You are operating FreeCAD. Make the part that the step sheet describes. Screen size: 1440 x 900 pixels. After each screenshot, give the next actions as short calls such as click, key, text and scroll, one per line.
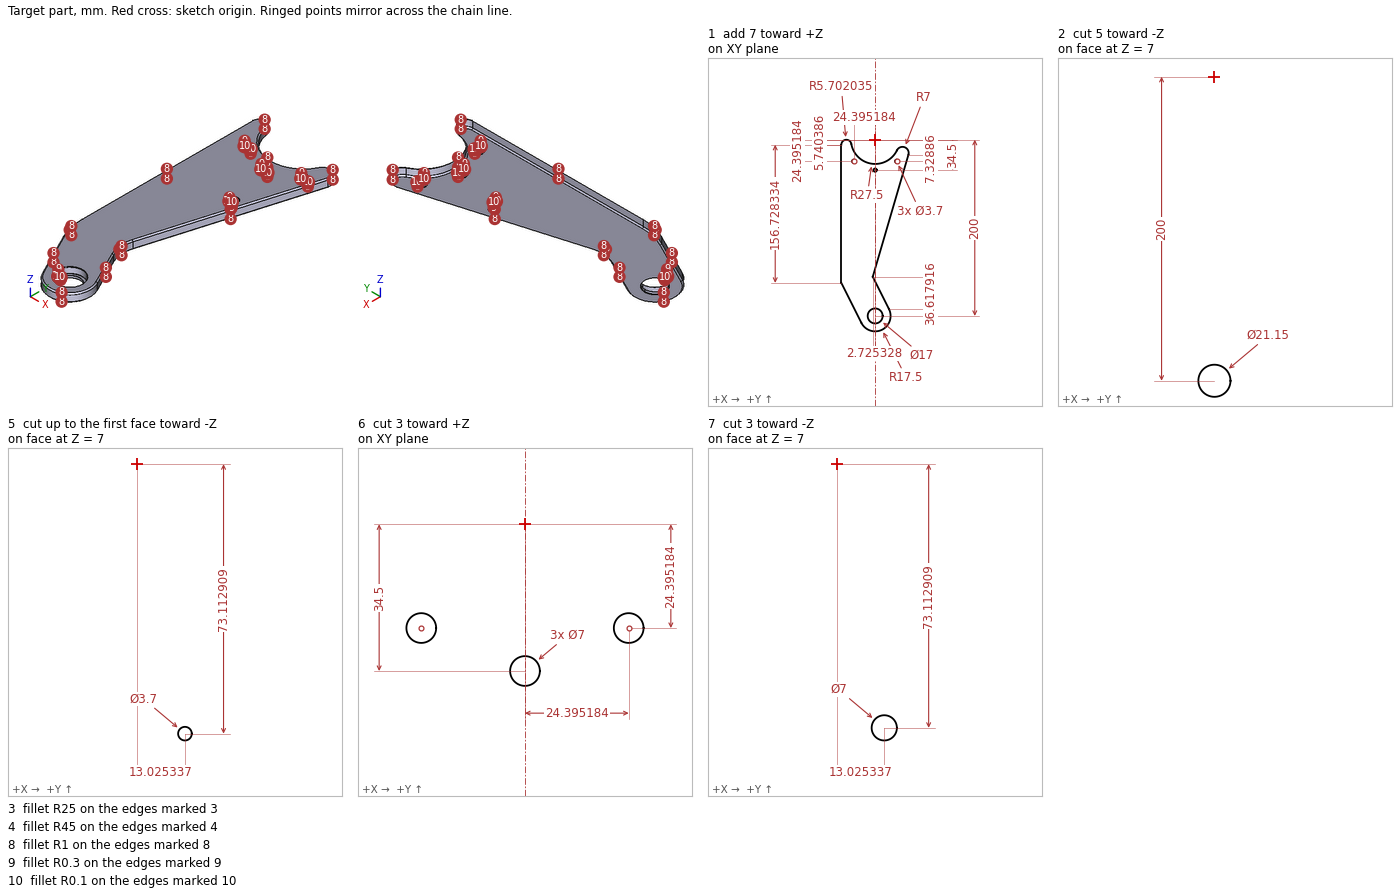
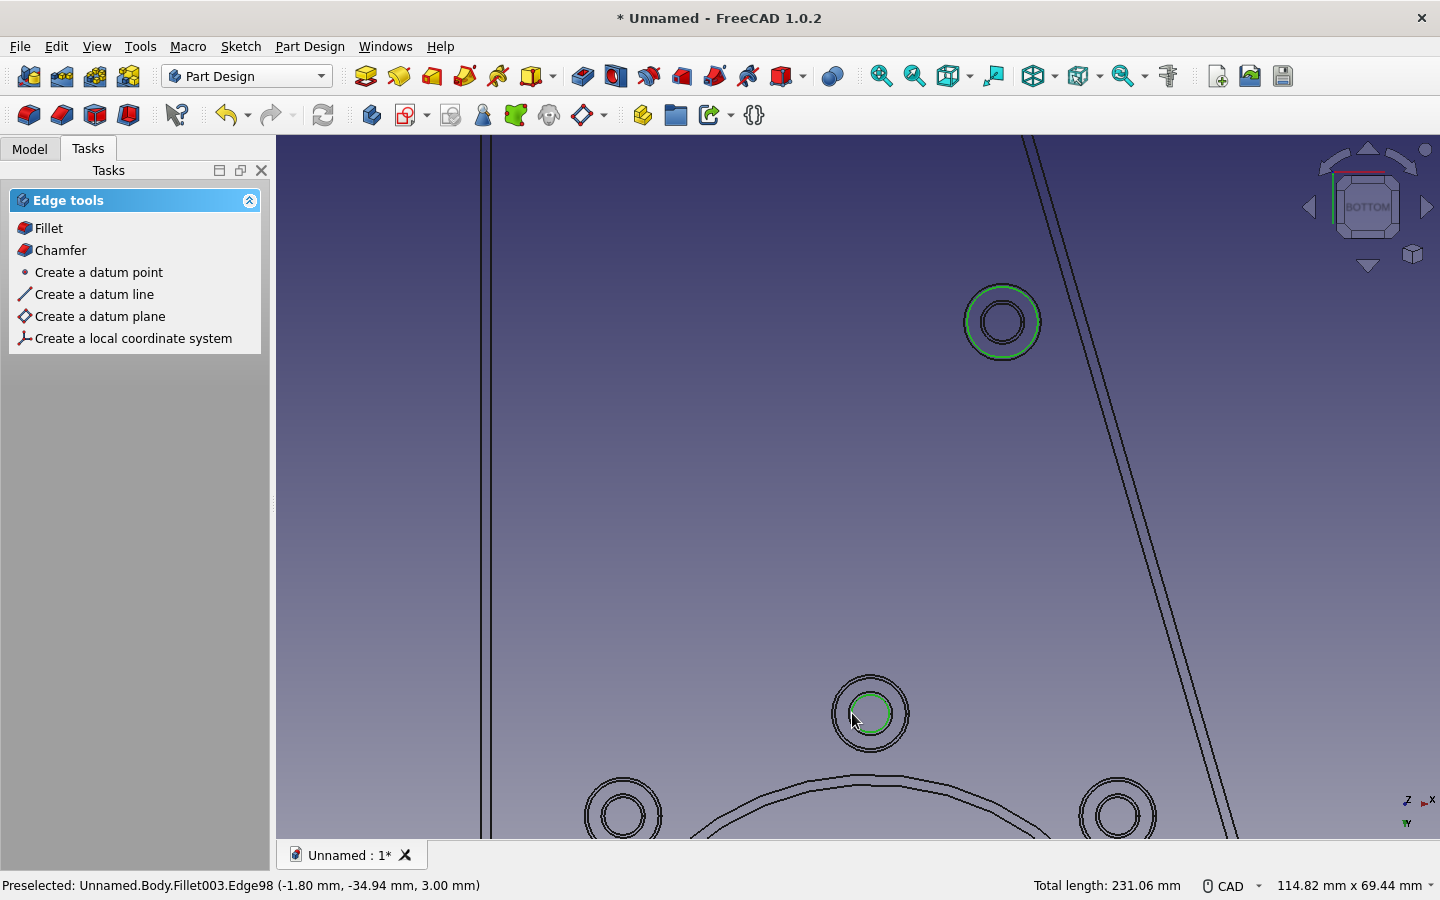
click(1103, 804, ctrl)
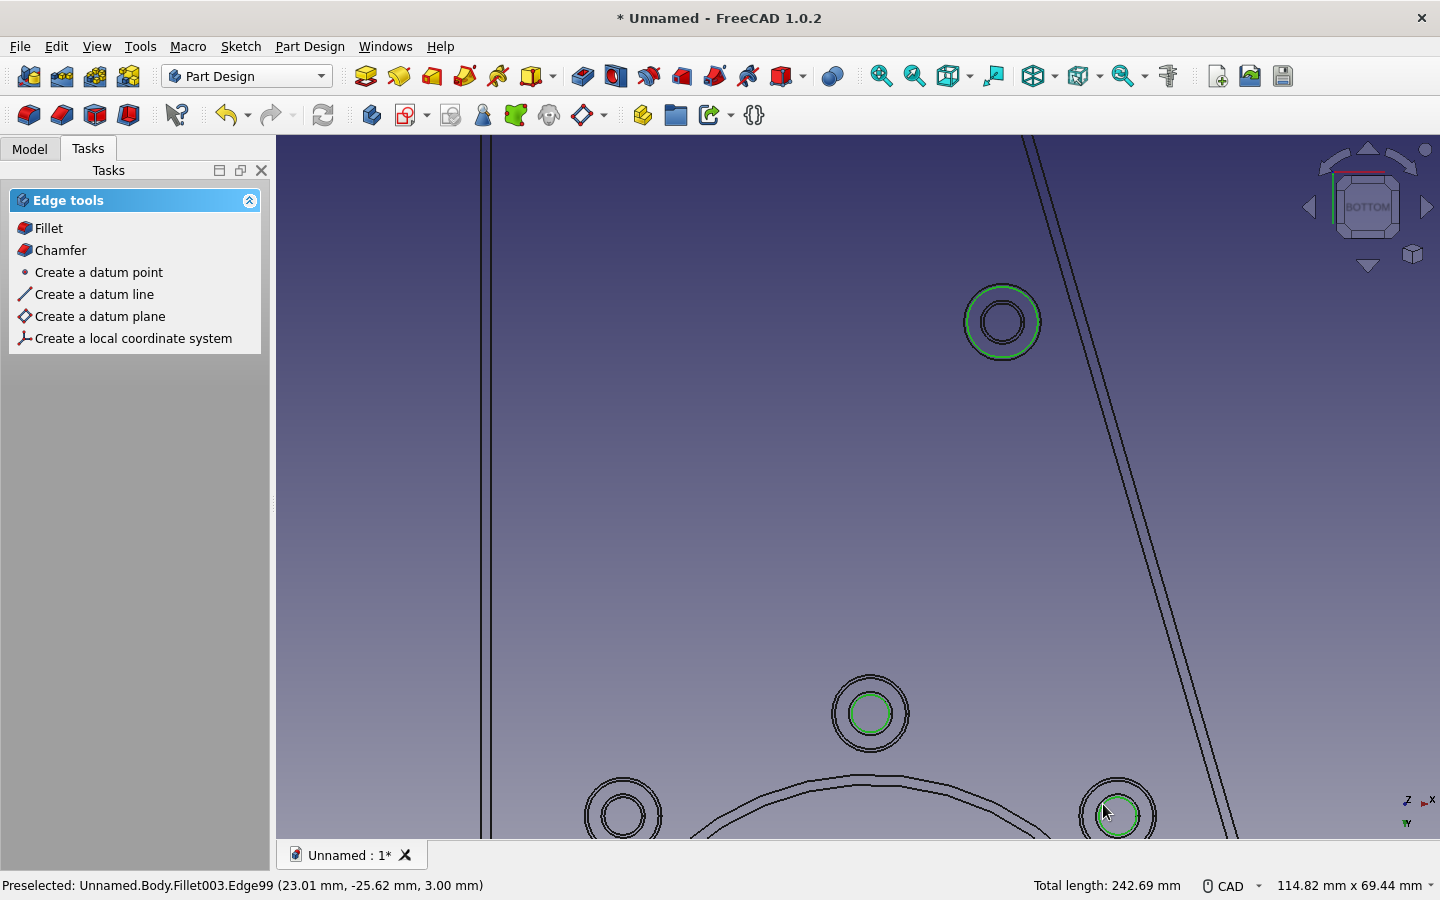
click(608, 804, ctrl)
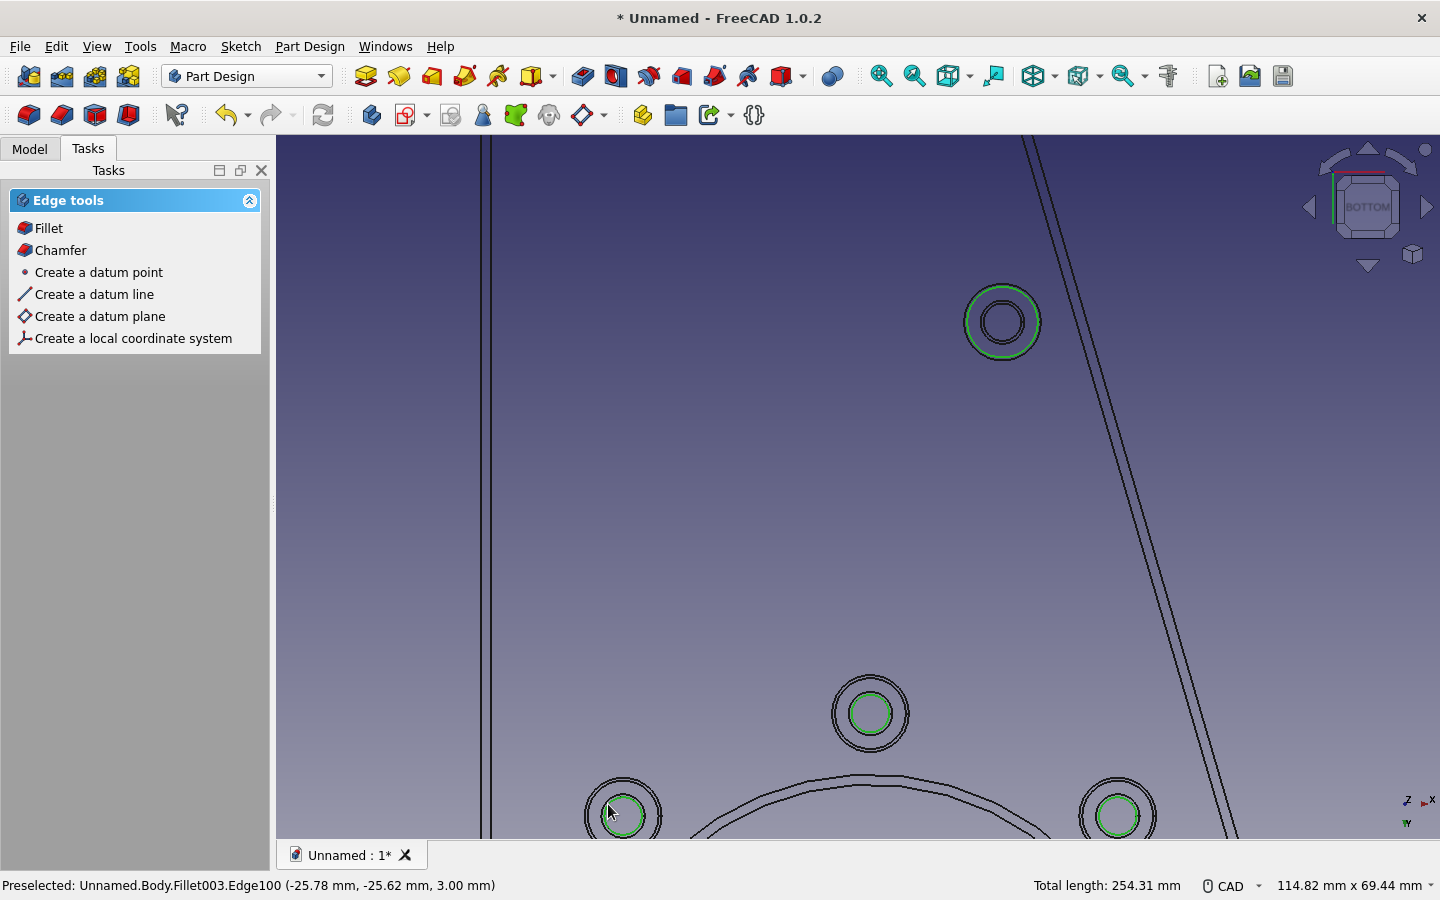
key(v)
key(1)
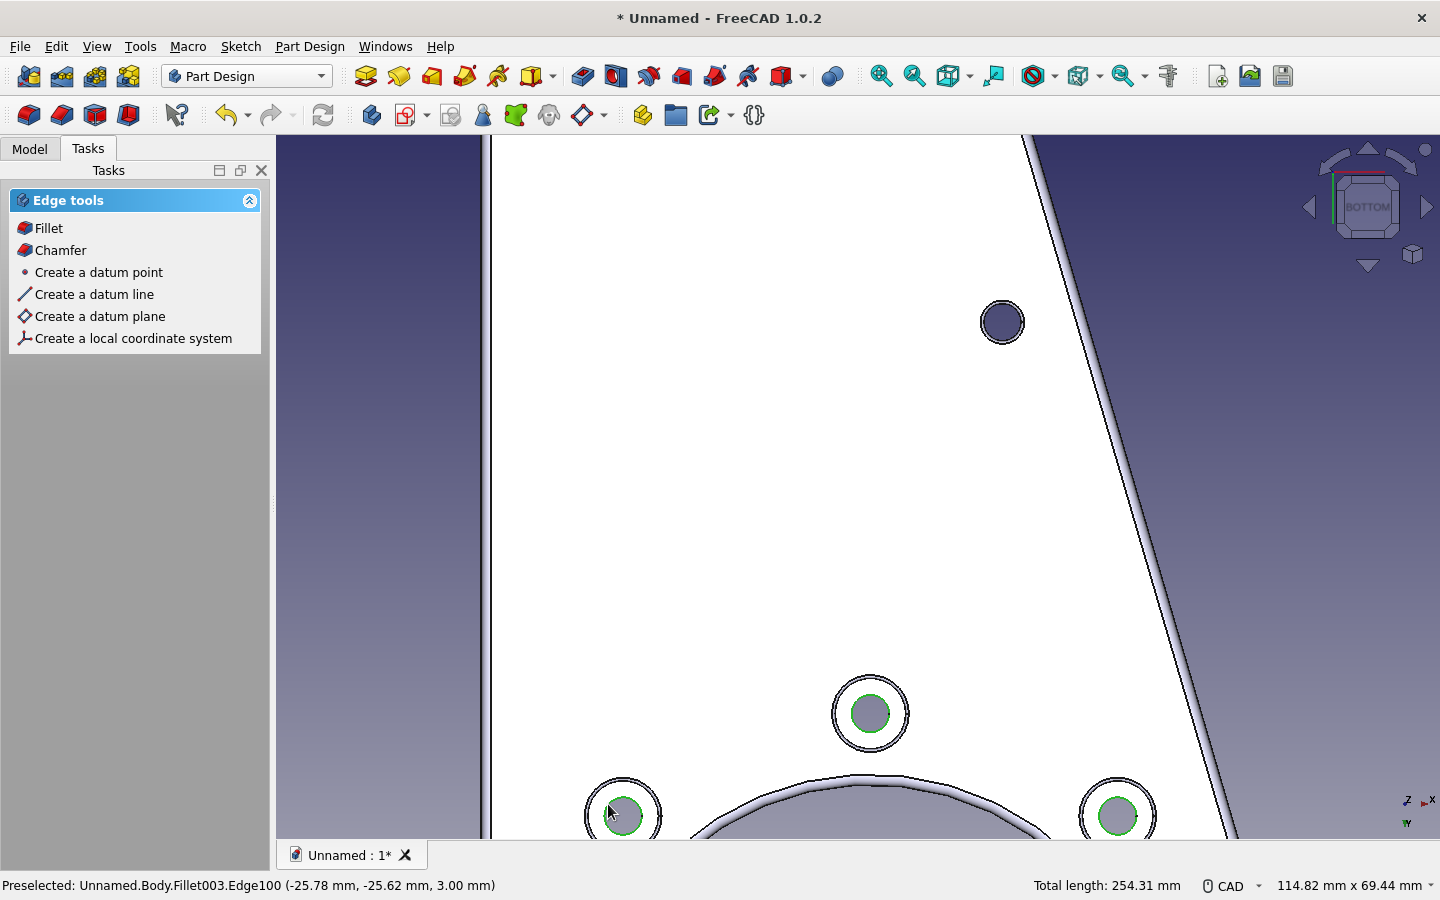
click(29, 116)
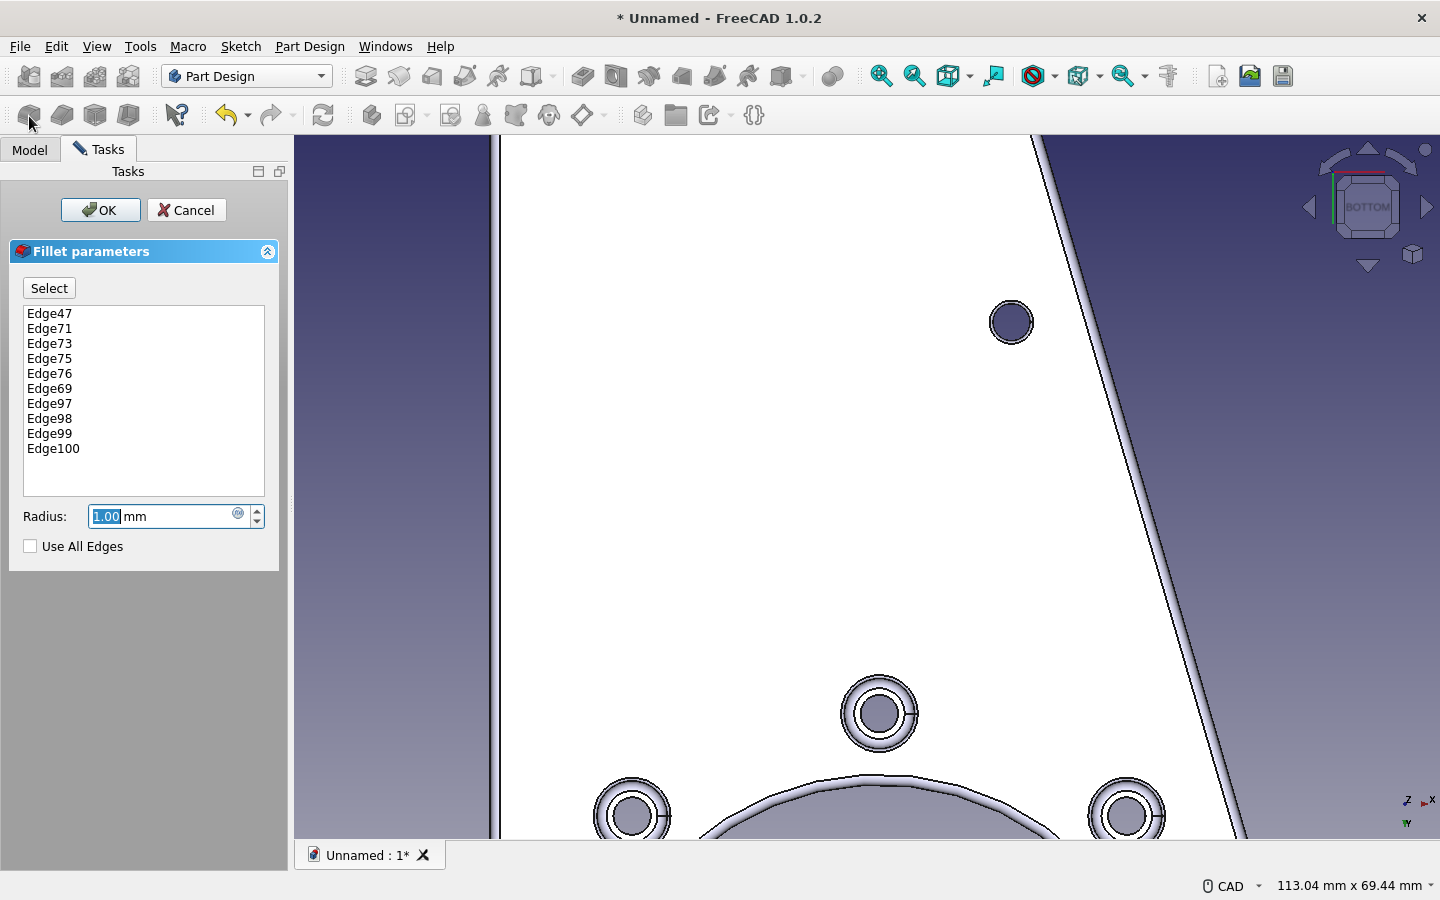
text(0.1)
key(Tab)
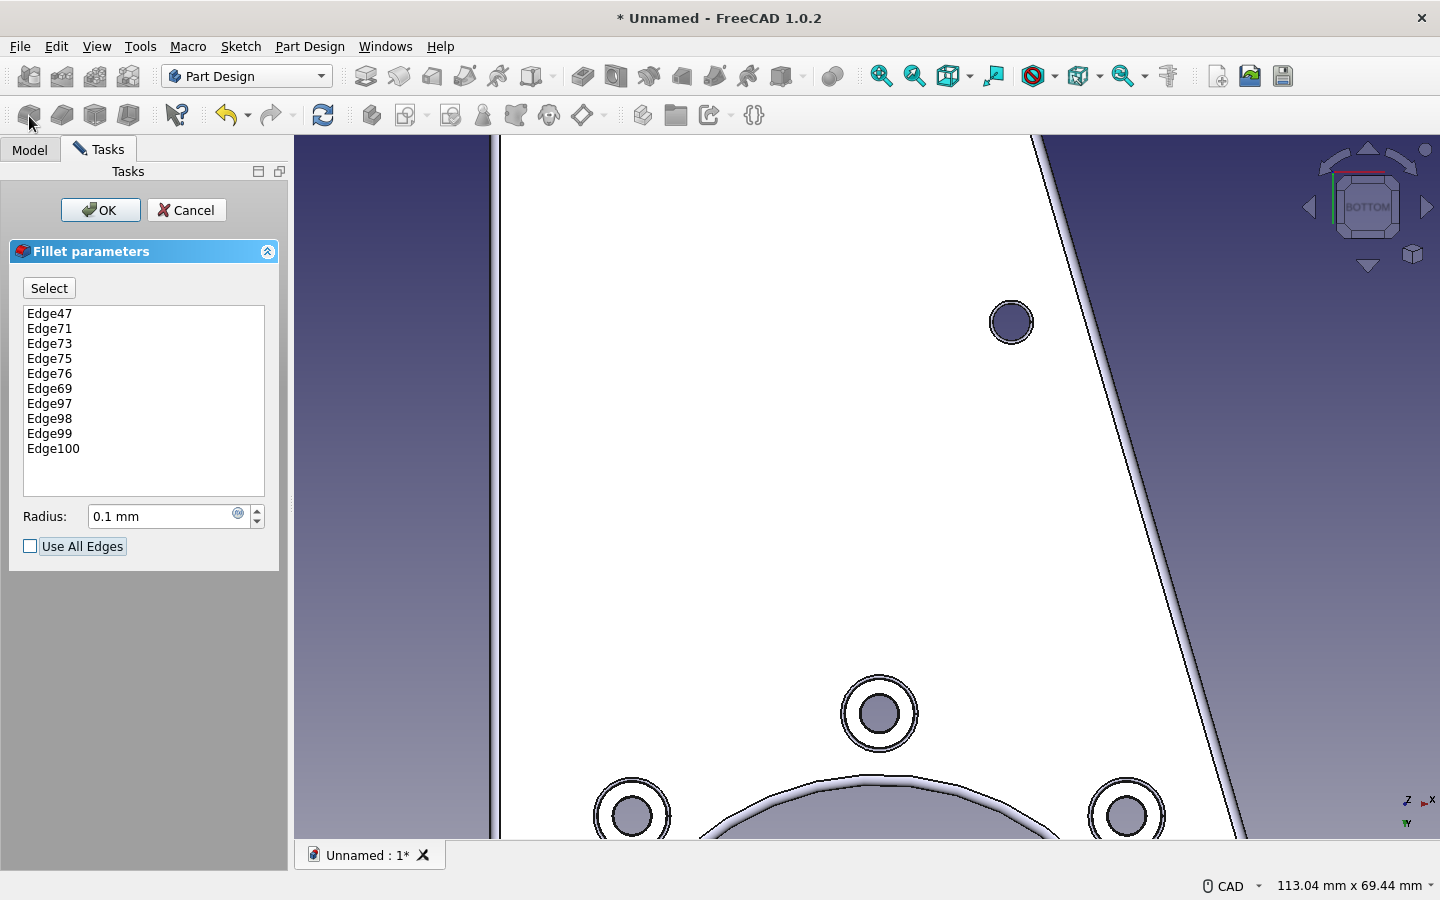
click(101, 210)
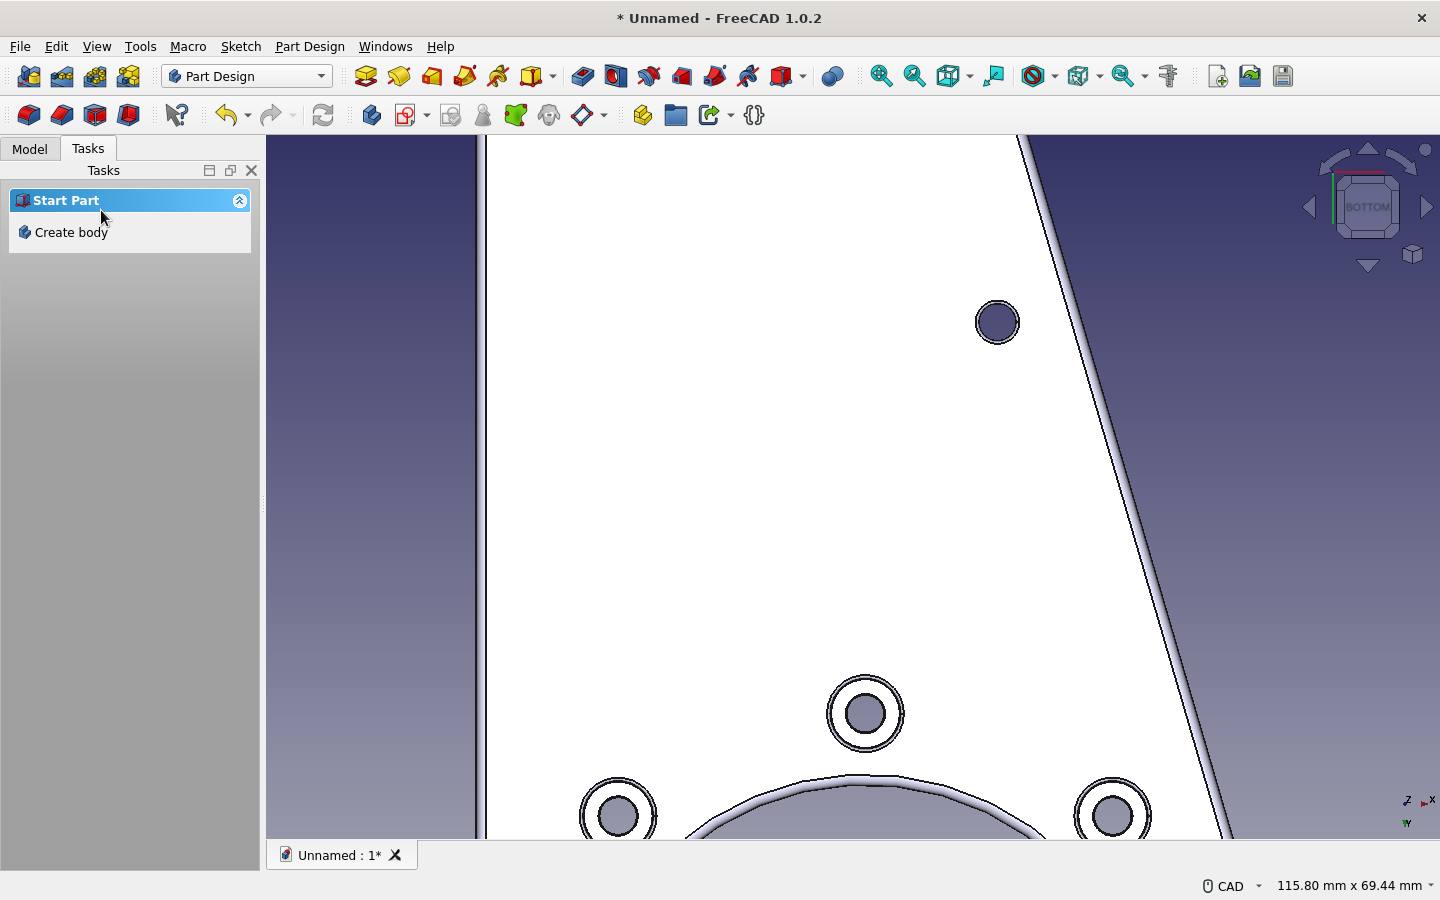
key(0)